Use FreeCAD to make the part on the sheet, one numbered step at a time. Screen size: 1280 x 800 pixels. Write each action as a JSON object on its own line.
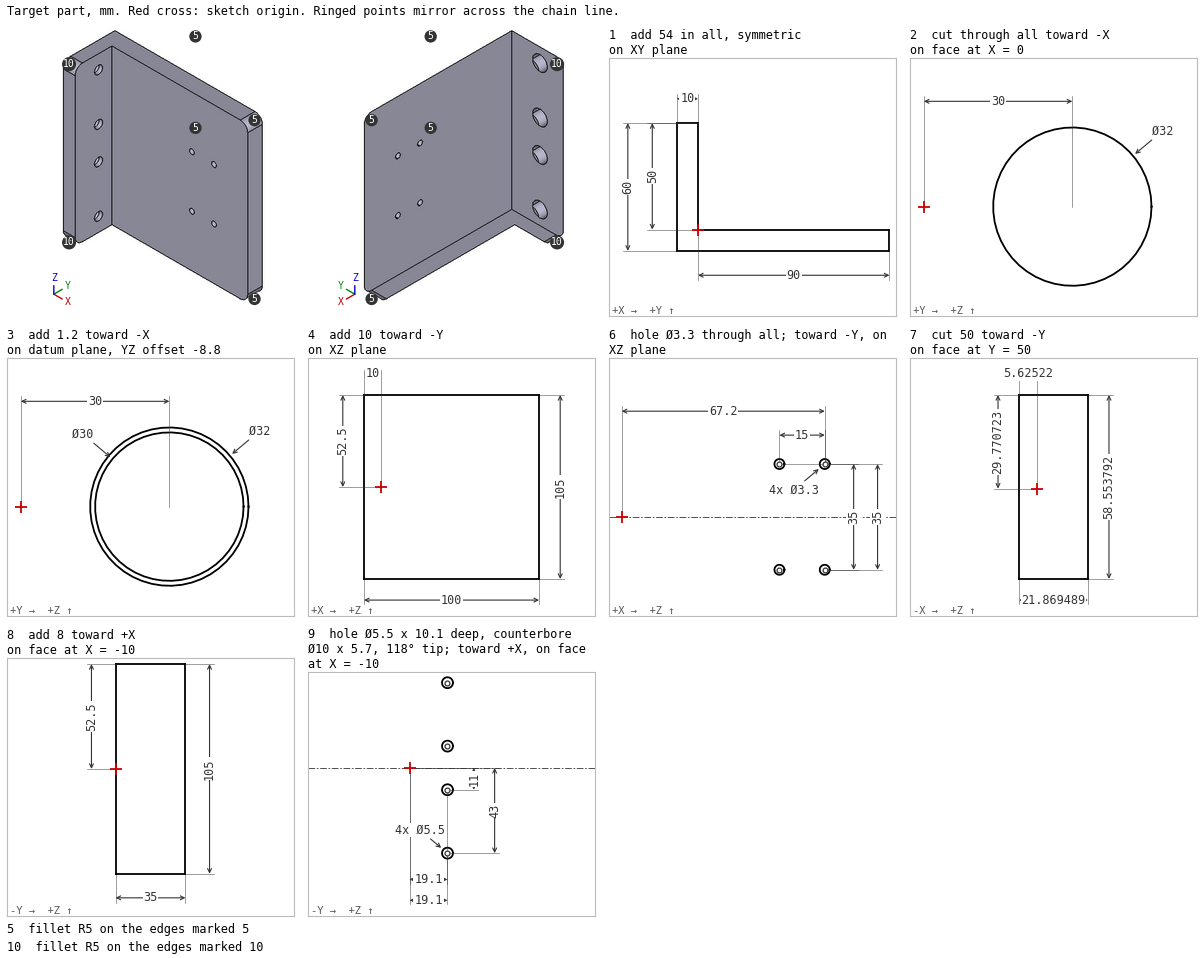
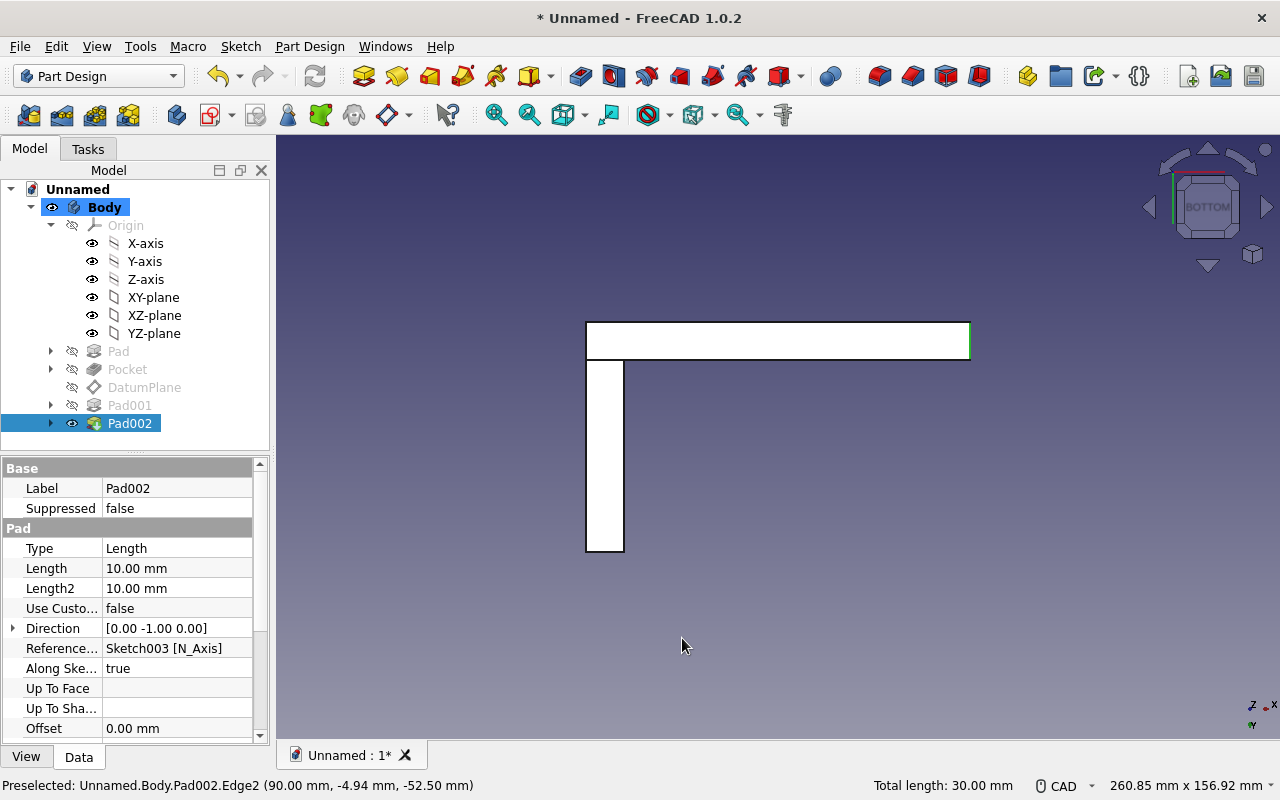
{"action": "left_click", "coordinate": [497, 116]}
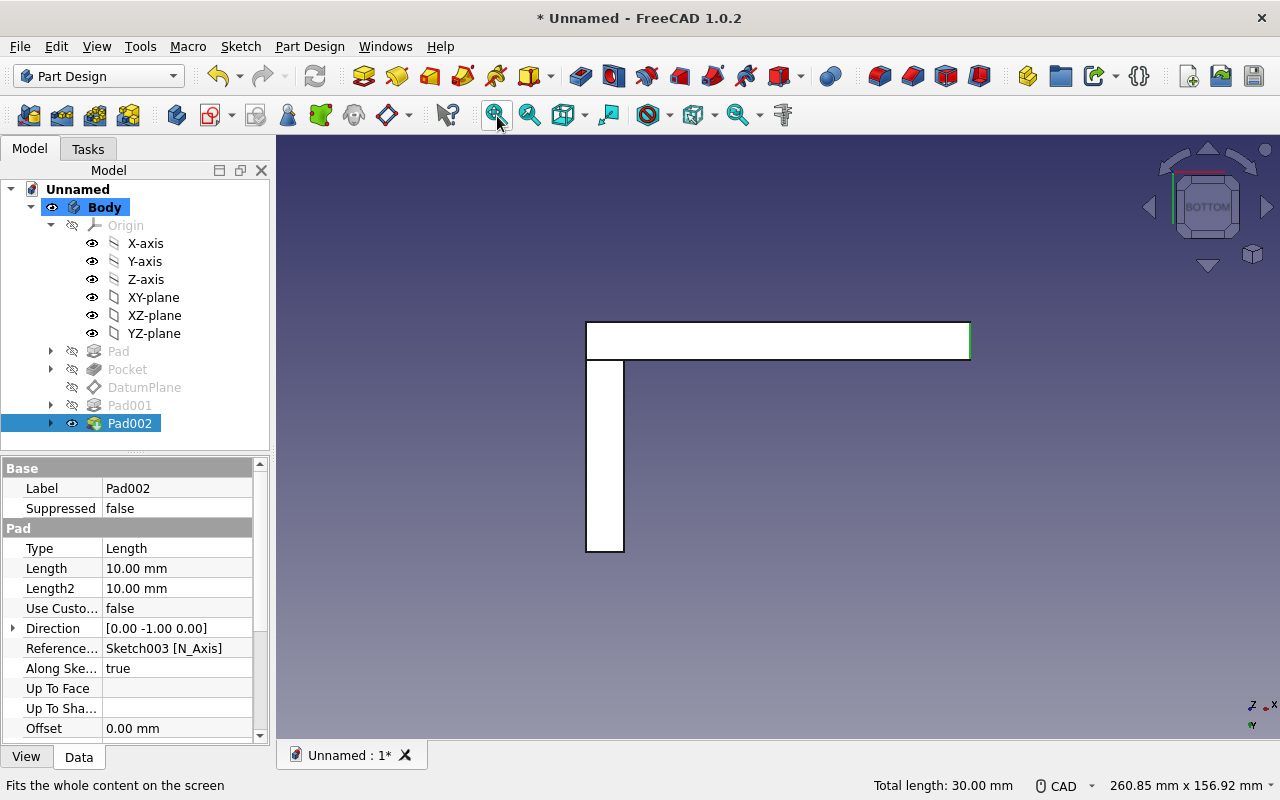
{"action": "left_click", "coordinate": [605, 551], "text": "ctrl"}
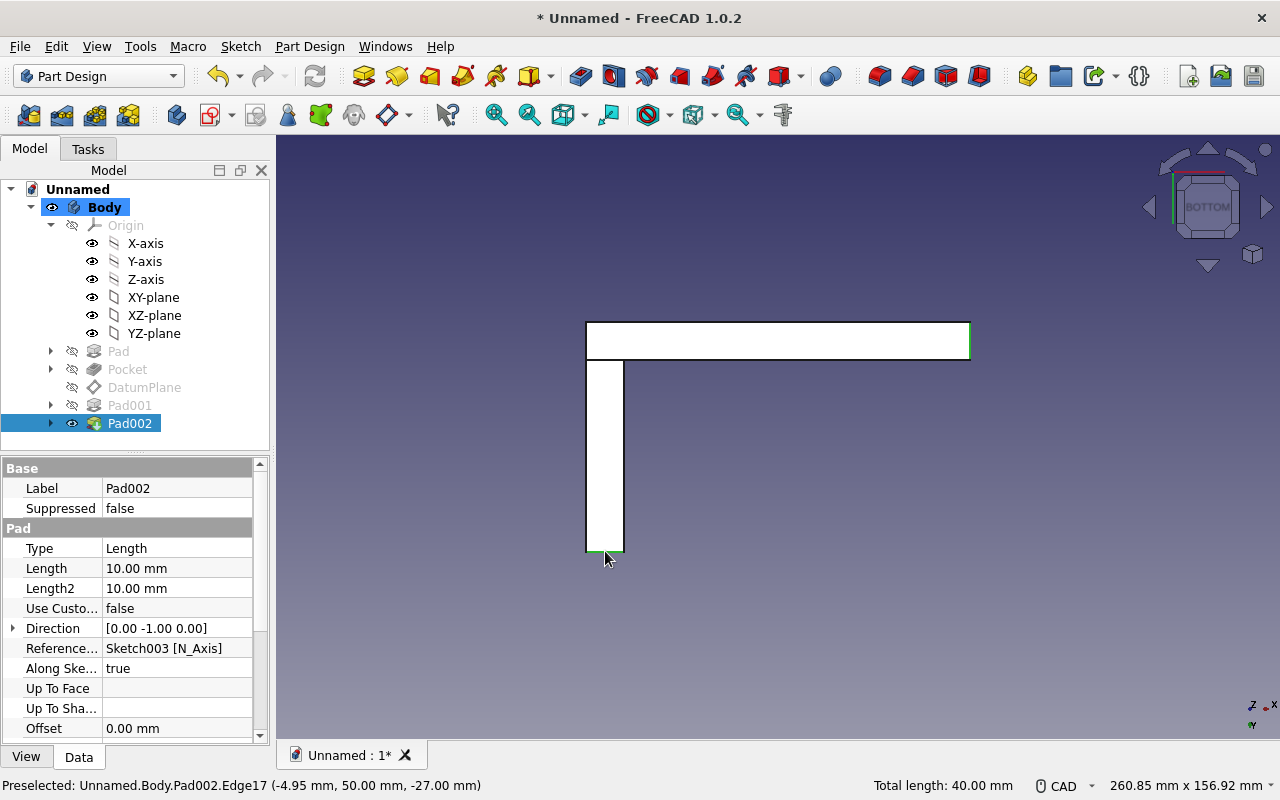
{"action": "left_click", "coordinate": [880, 76]}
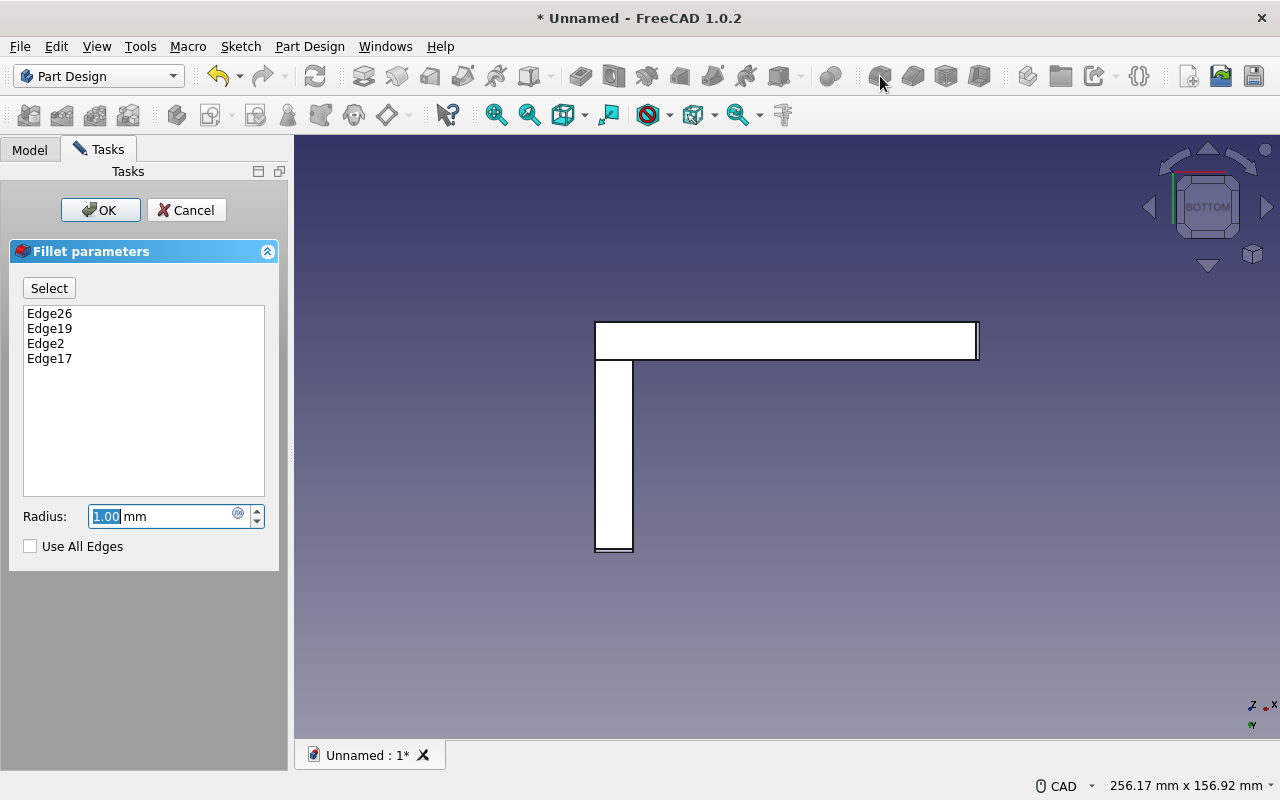
{"action": "type", "text": "5"}
{"action": "key", "text": "Tab"}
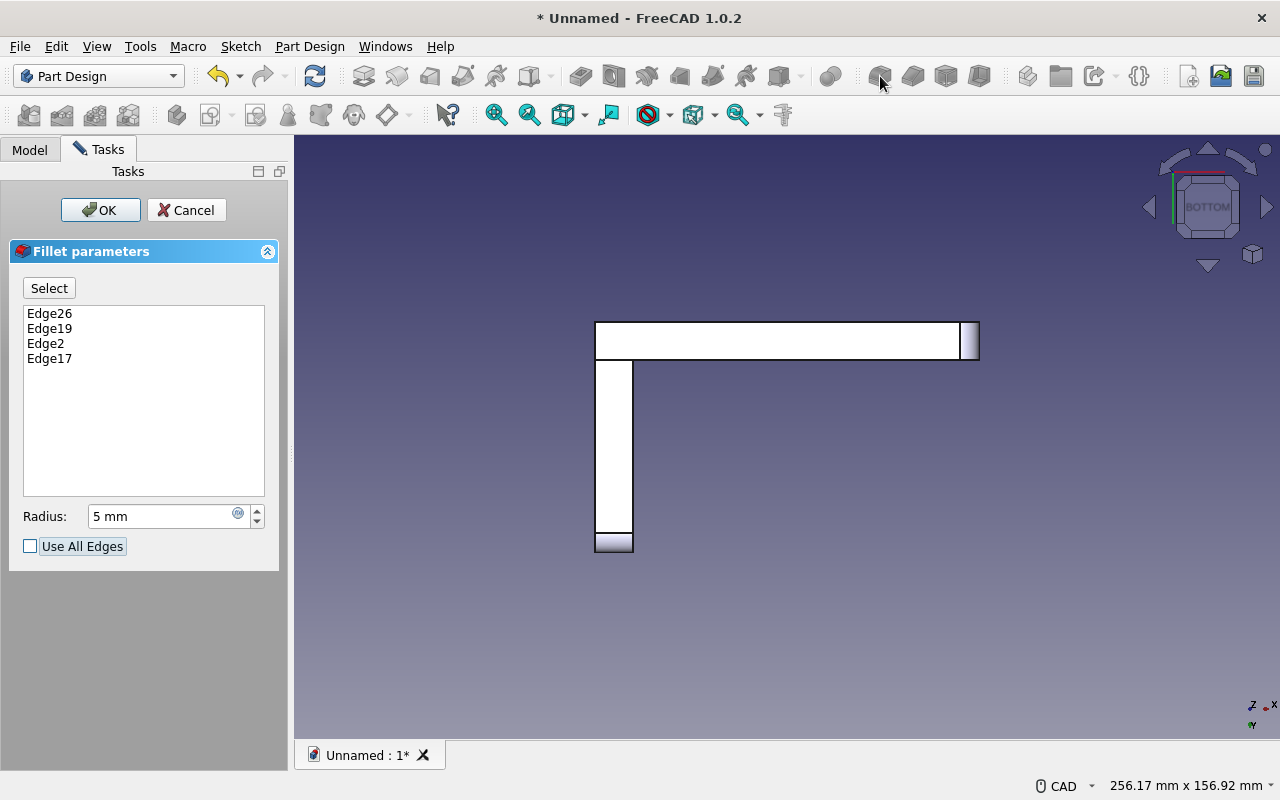
{"action": "left_click", "coordinate": [101, 210]}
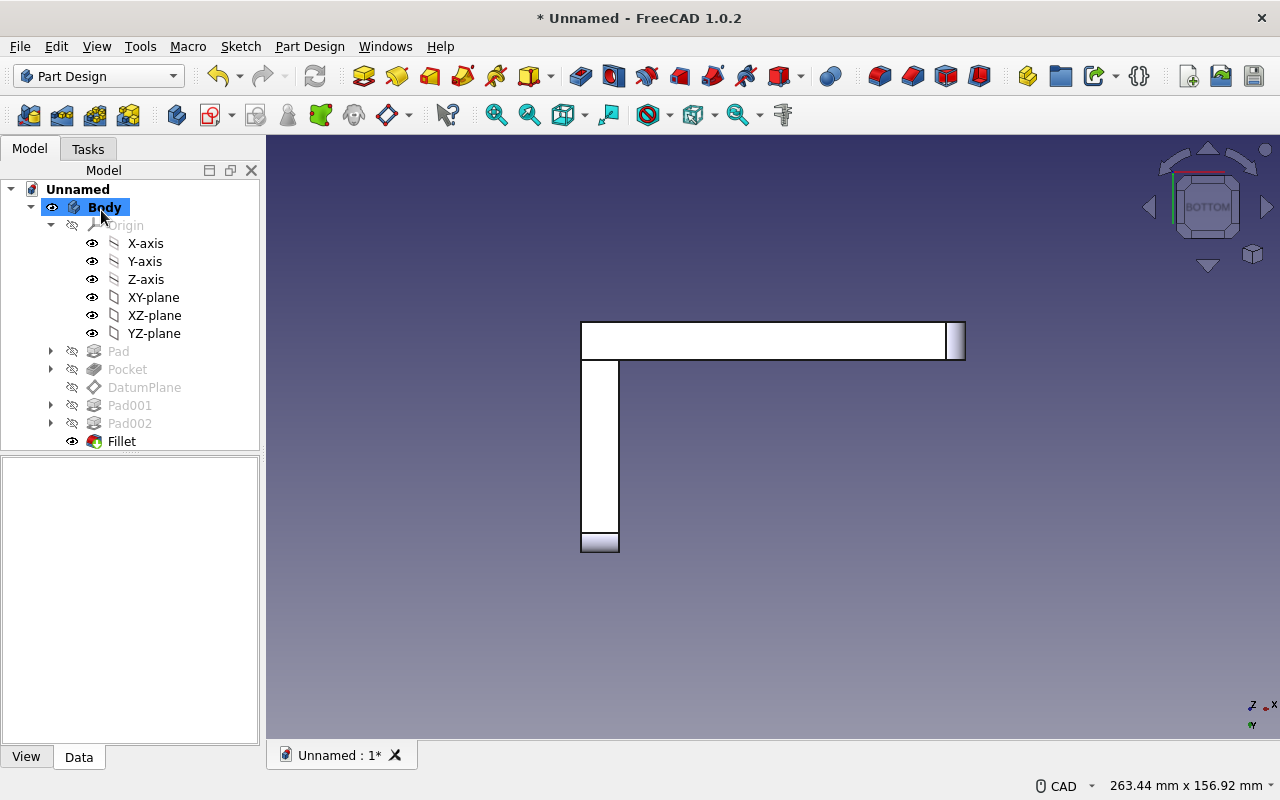
{"action": "left_click", "coordinate": [497, 116]}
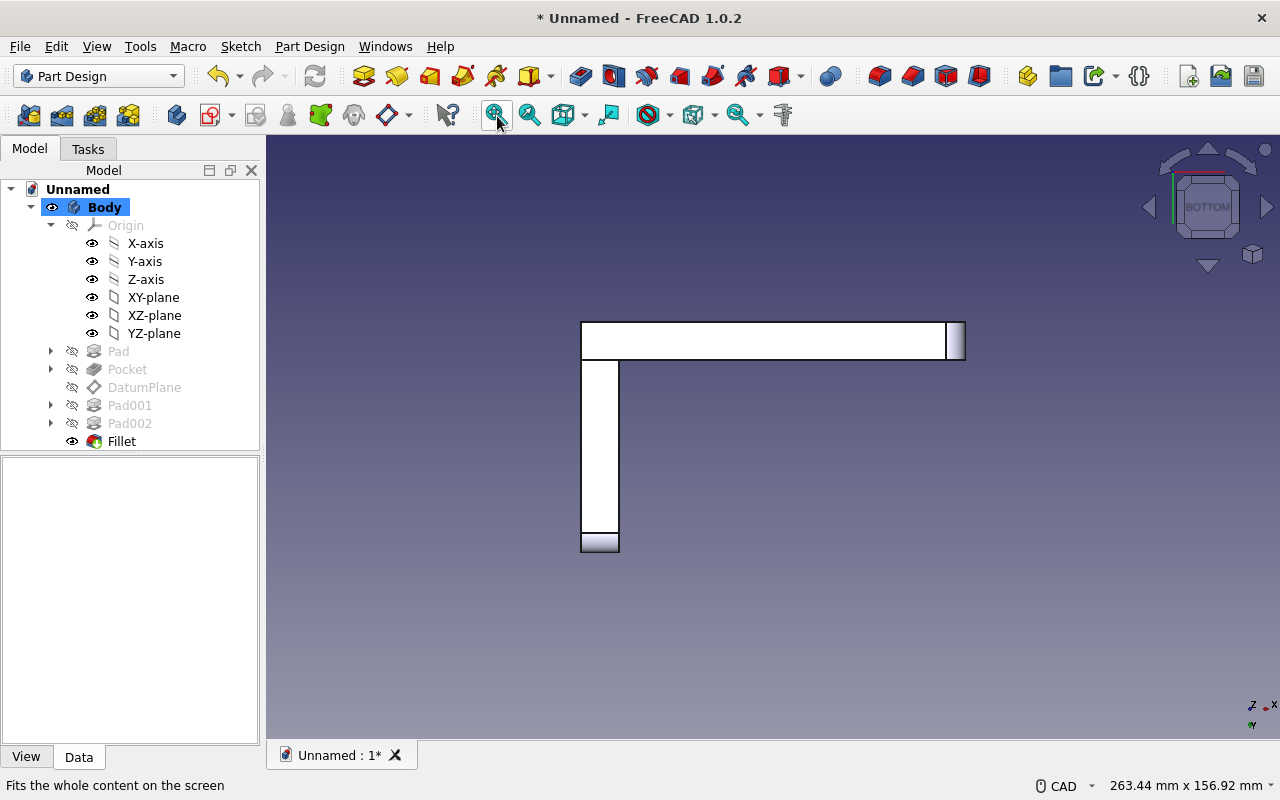
{"action": "left_click", "coordinate": [210, 116]}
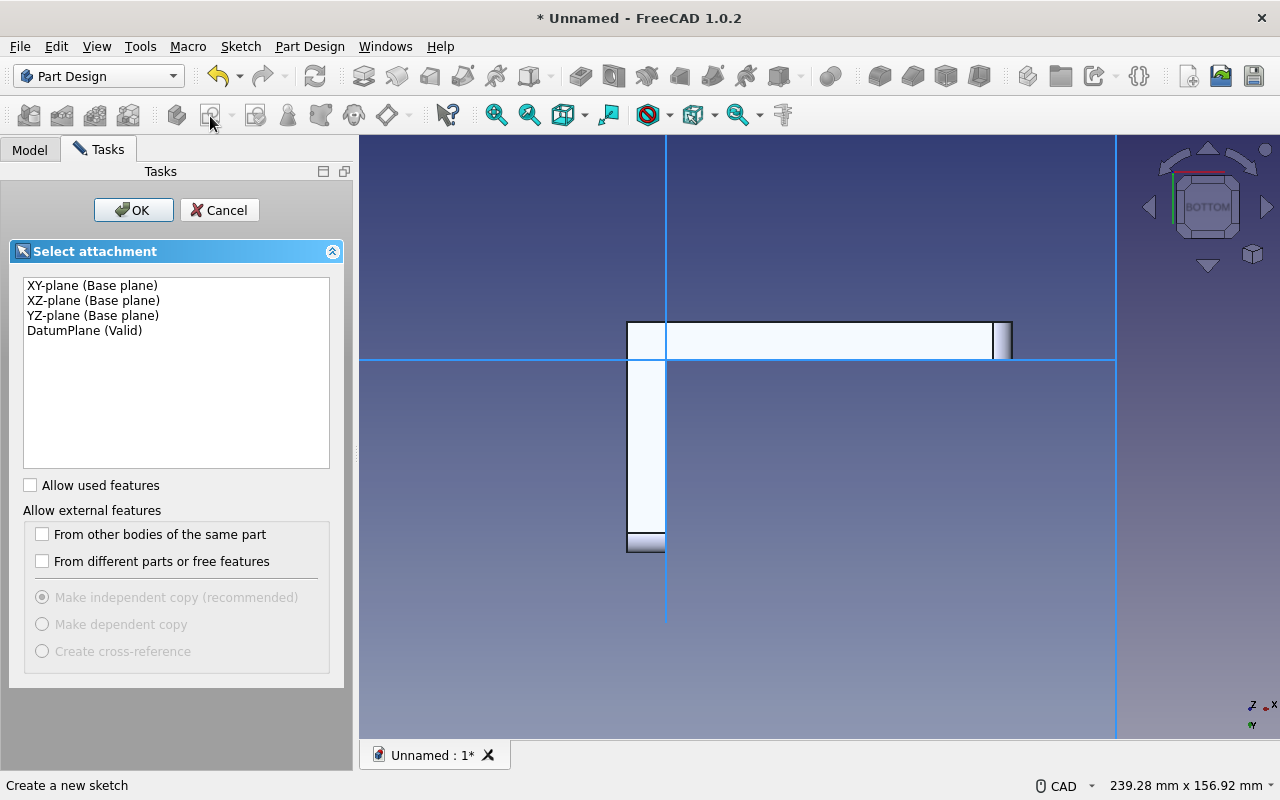
{"action": "left_click", "coordinate": [84, 300]}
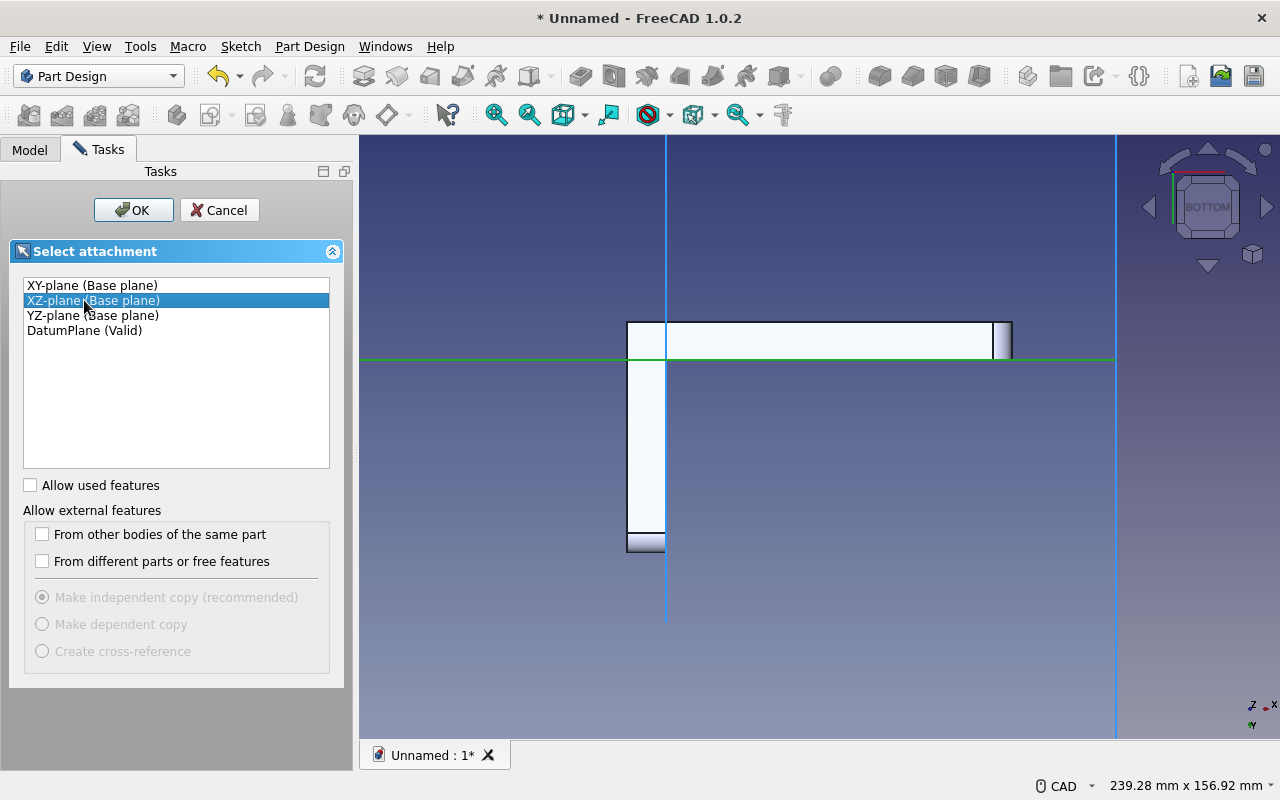
{"action": "left_click", "coordinate": [134, 210]}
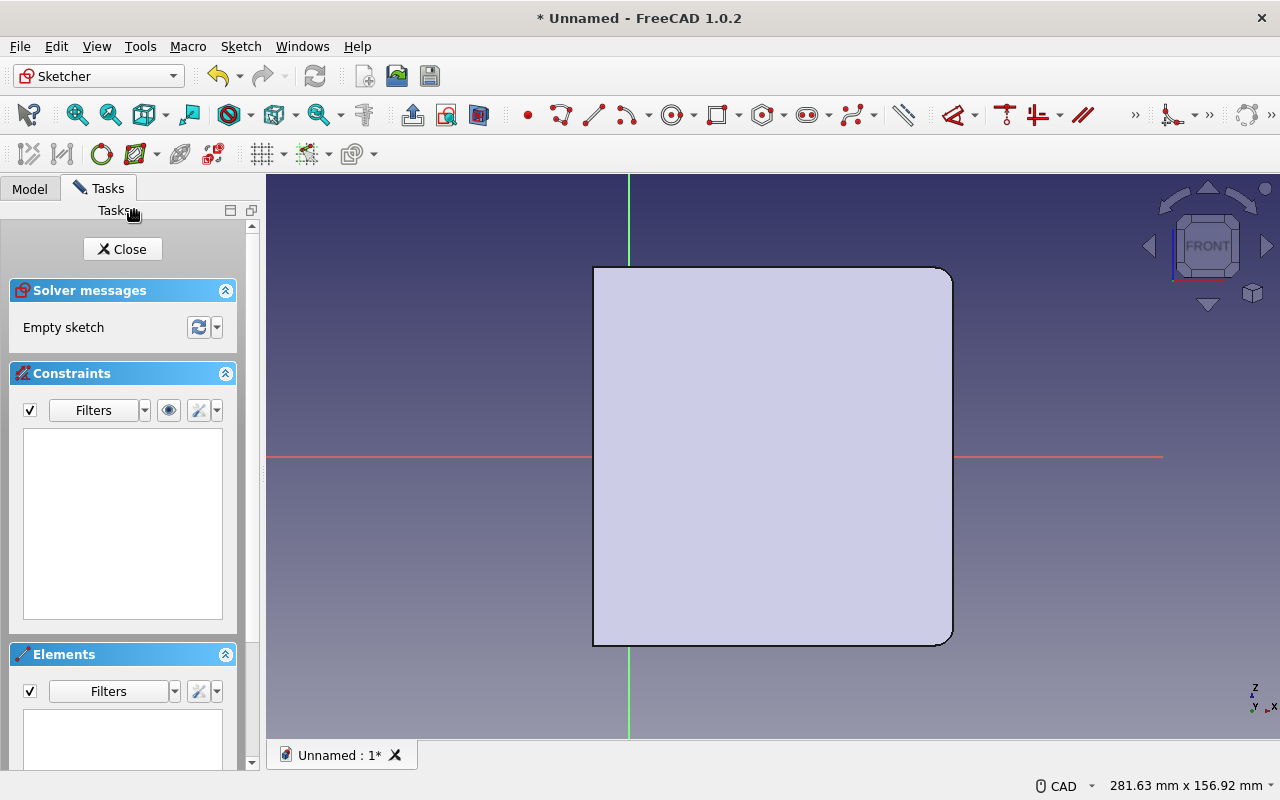
{"action": "left_click", "coordinate": [479, 116]}